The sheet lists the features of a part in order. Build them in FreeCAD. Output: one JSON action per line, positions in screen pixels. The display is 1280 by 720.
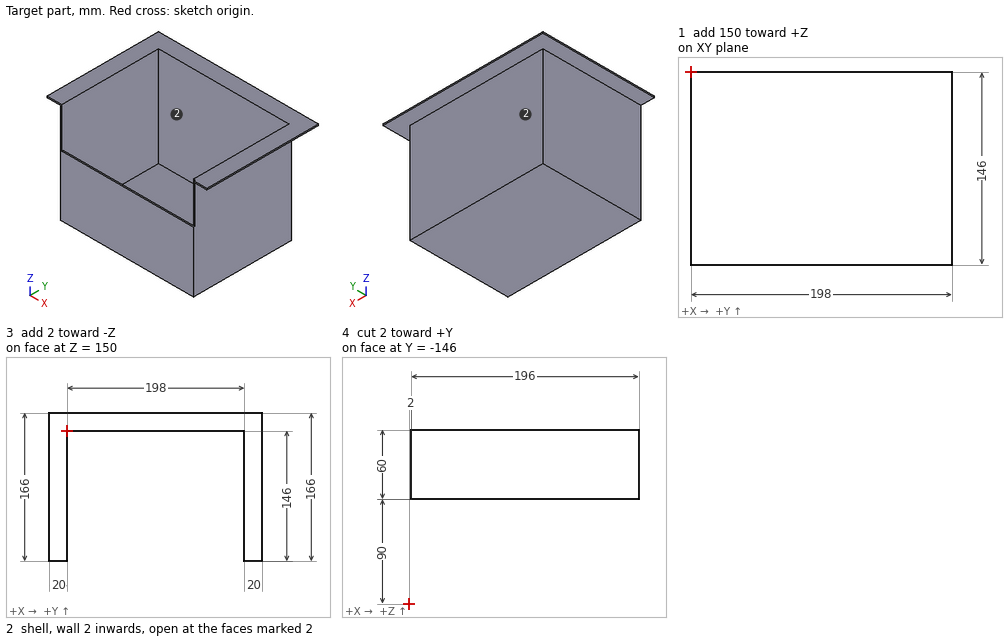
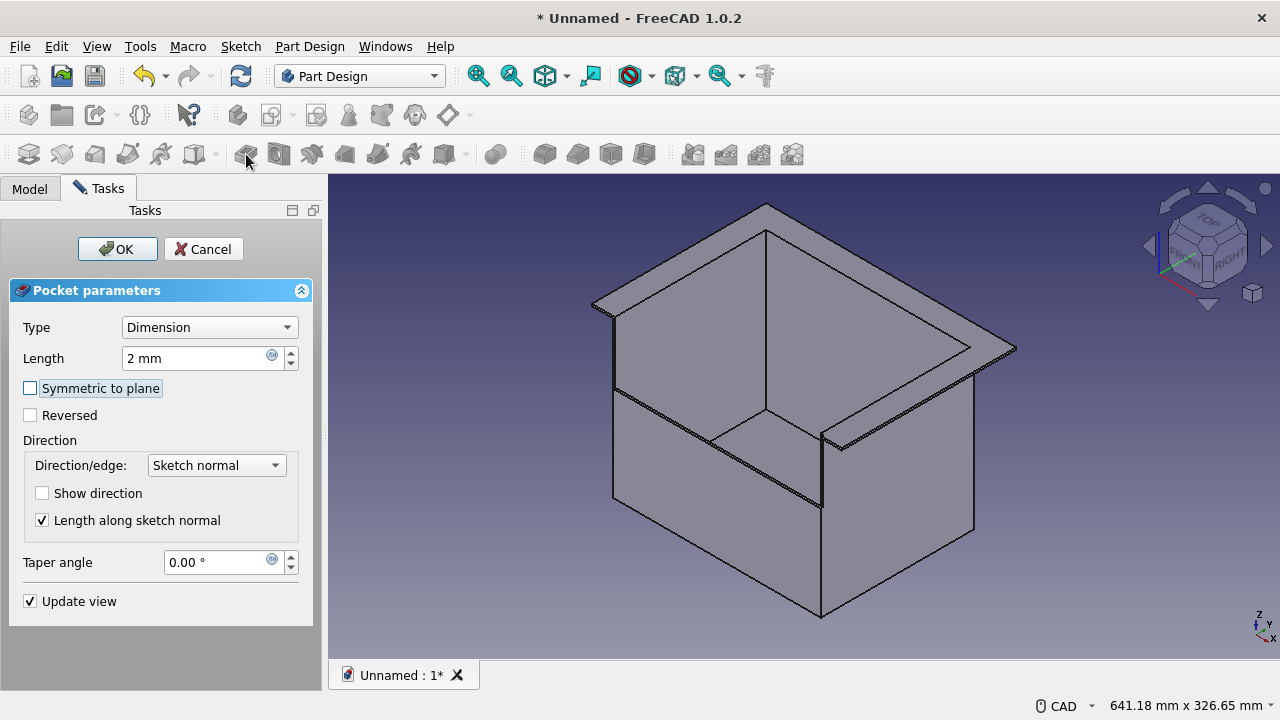
{"action": "left_click", "coordinate": [118, 249]}